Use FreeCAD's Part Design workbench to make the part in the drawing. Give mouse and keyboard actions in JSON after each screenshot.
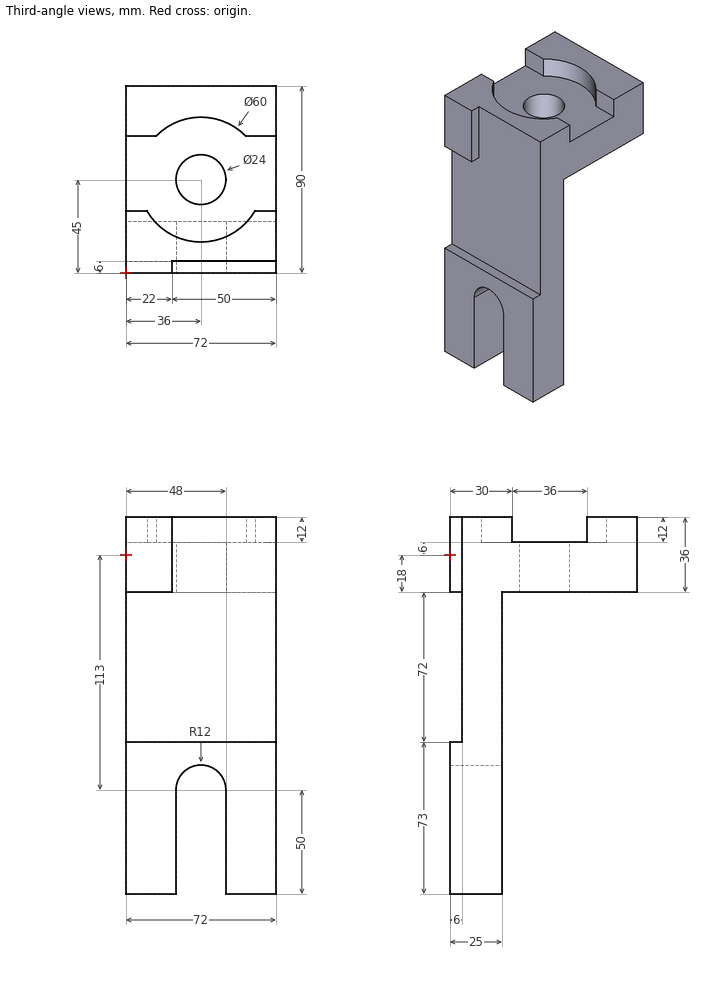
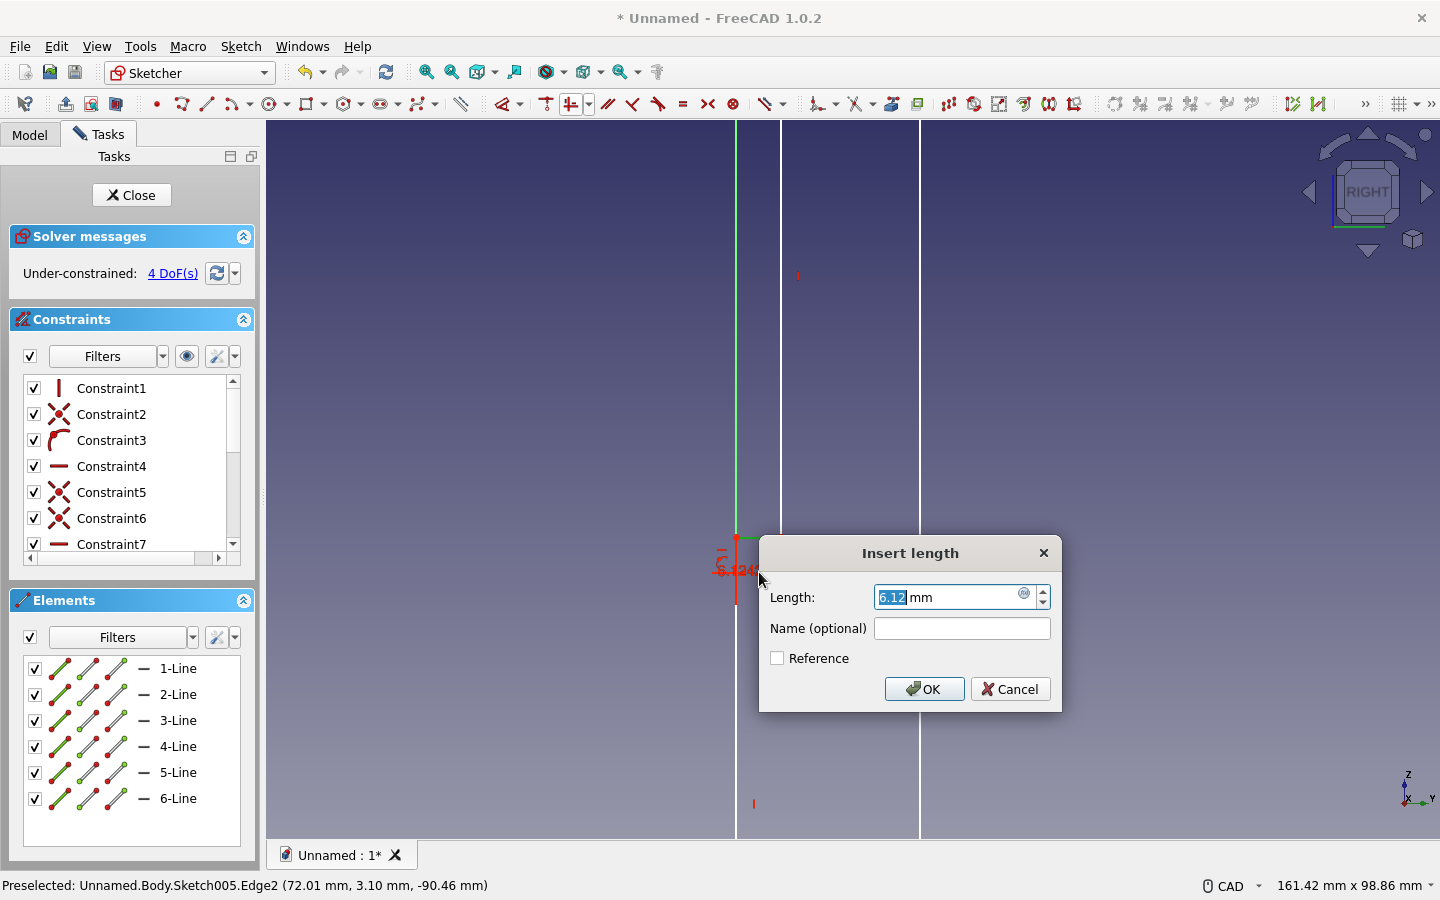
{"action": "type", "text": "6"}
{"action": "key", "text": "Return"}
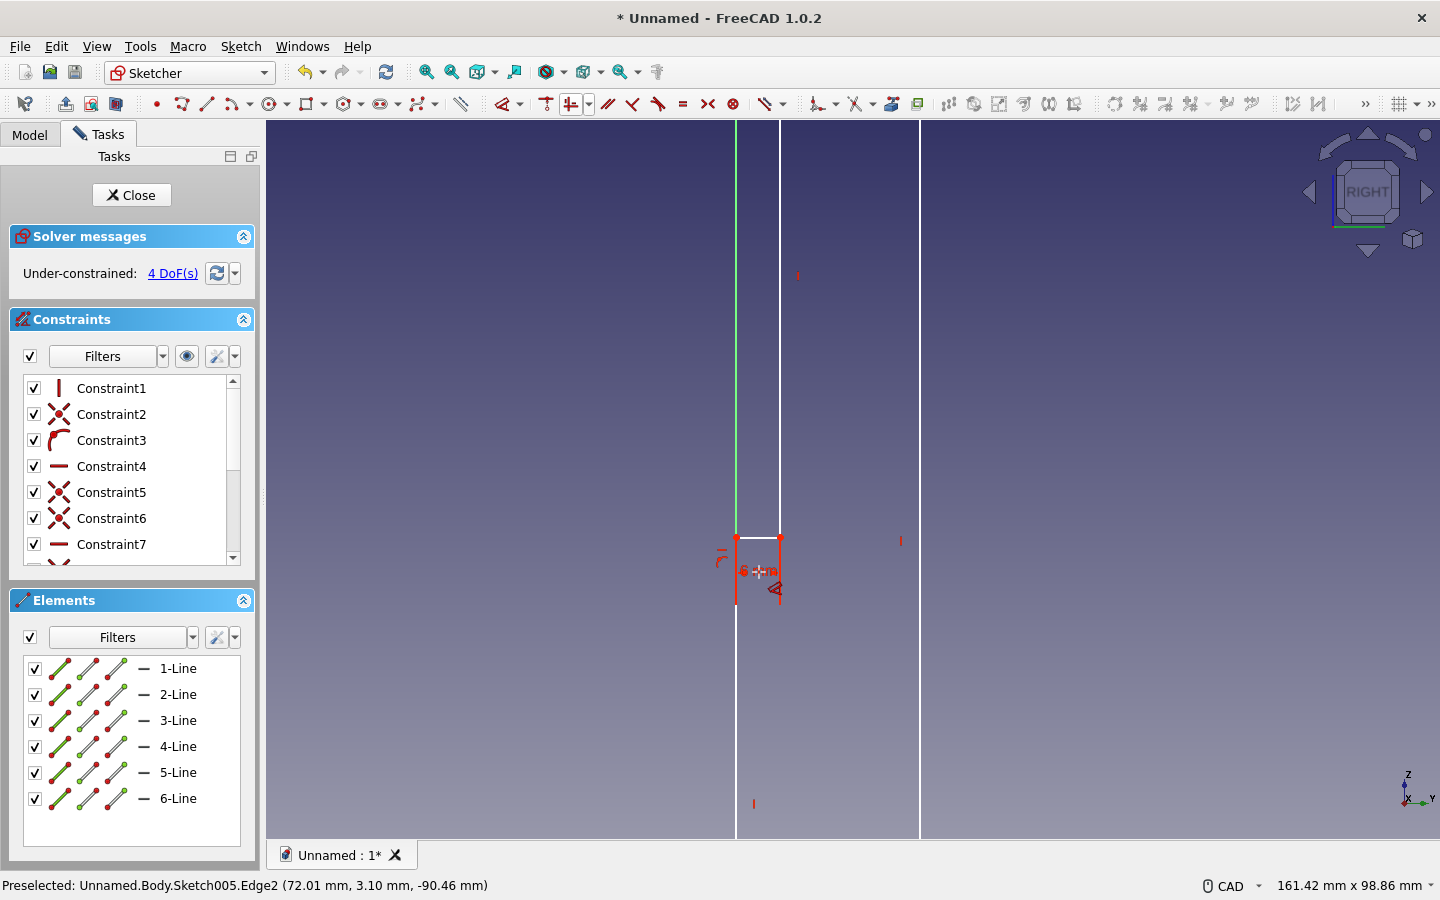
{"action": "left_click", "coordinate": [780, 171]}
{"action": "left_click", "coordinate": [814, 343]}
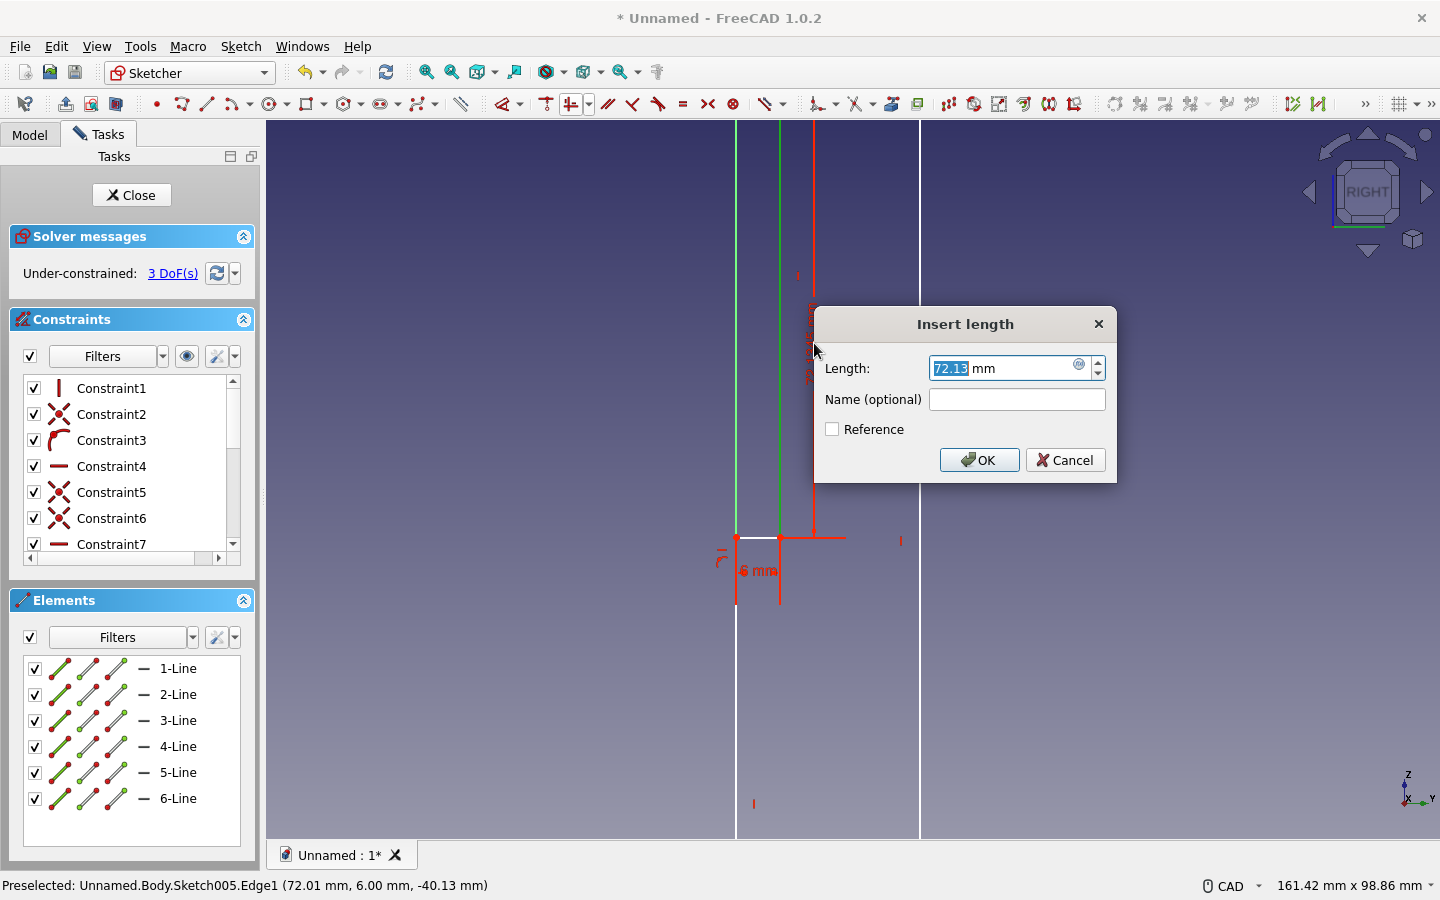
{"action": "type", "text": "72"}
{"action": "key", "text": "Return"}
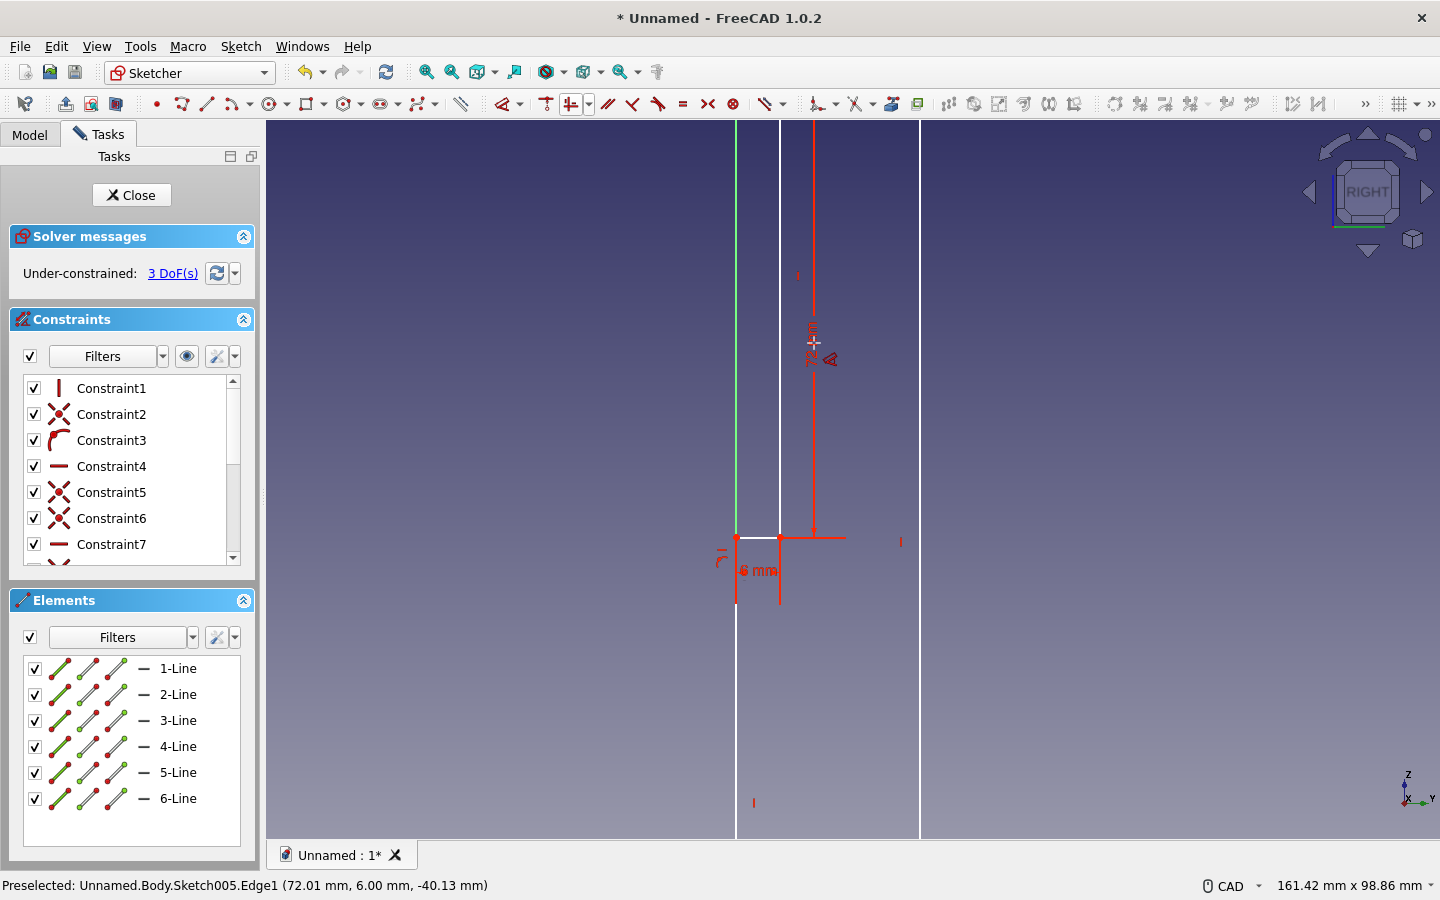
{"action": "left_click", "coordinate": [736, 697]}
{"action": "left_click", "coordinate": [702, 674]}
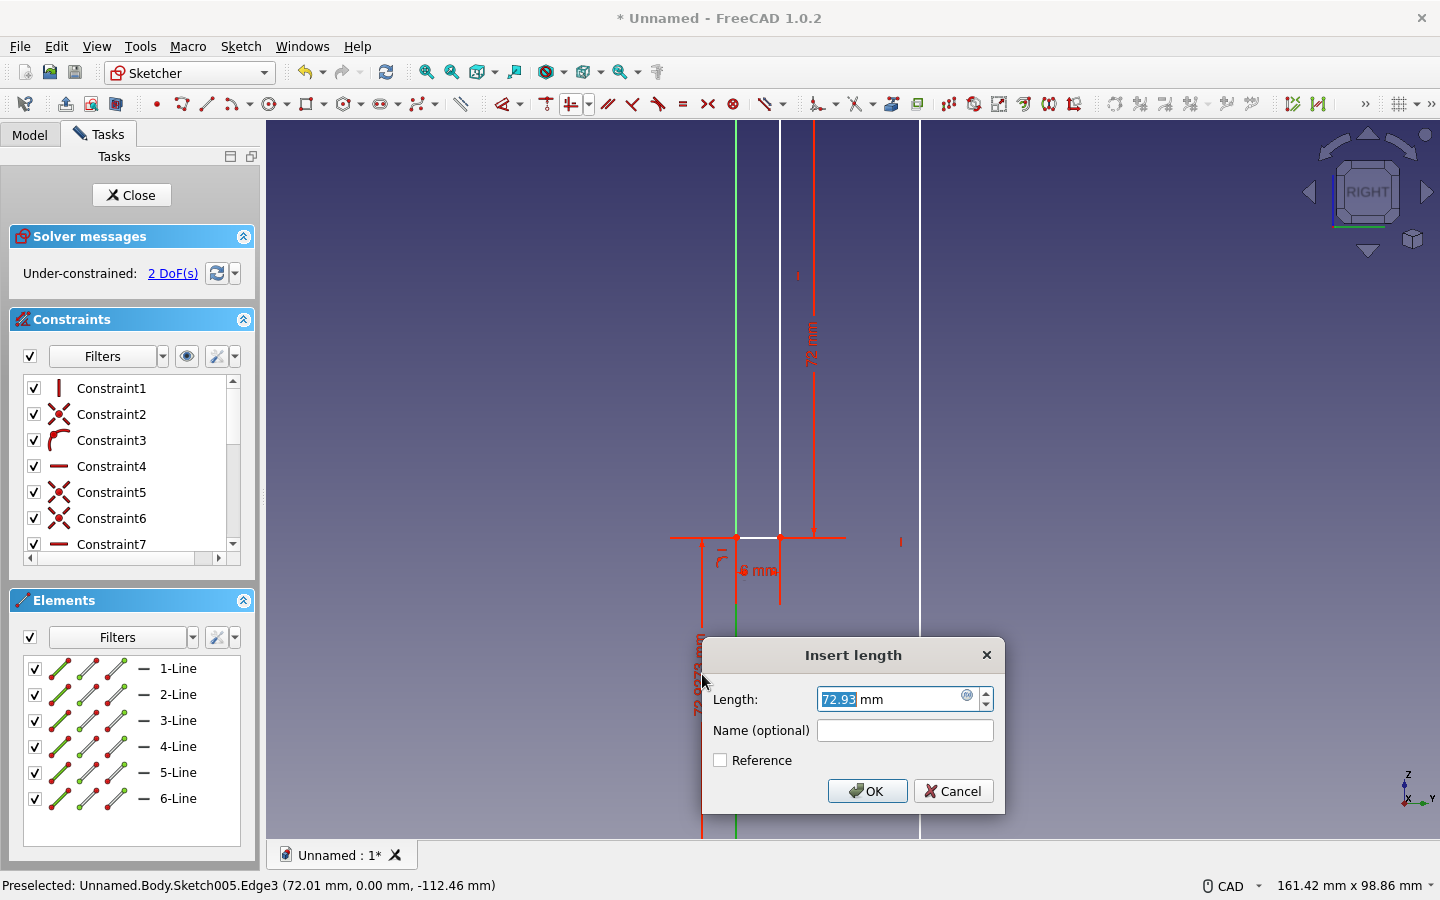
{"action": "type", "text": "73"}
{"action": "key", "text": "Return"}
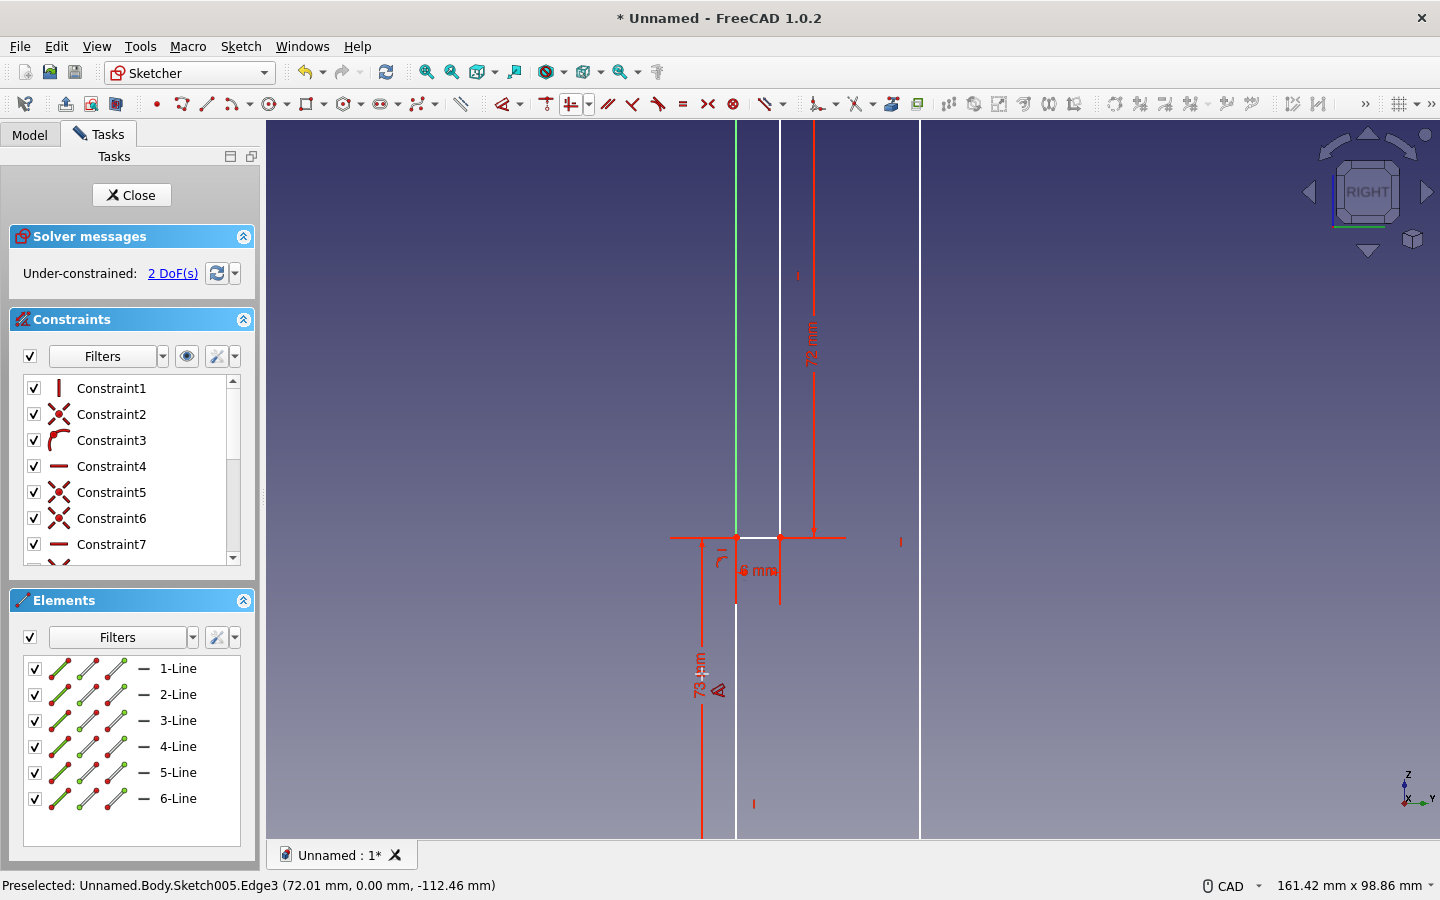
{"action": "scroll", "coordinate": [760, 483], "scroll_direction": "down", "scroll_amount": 5}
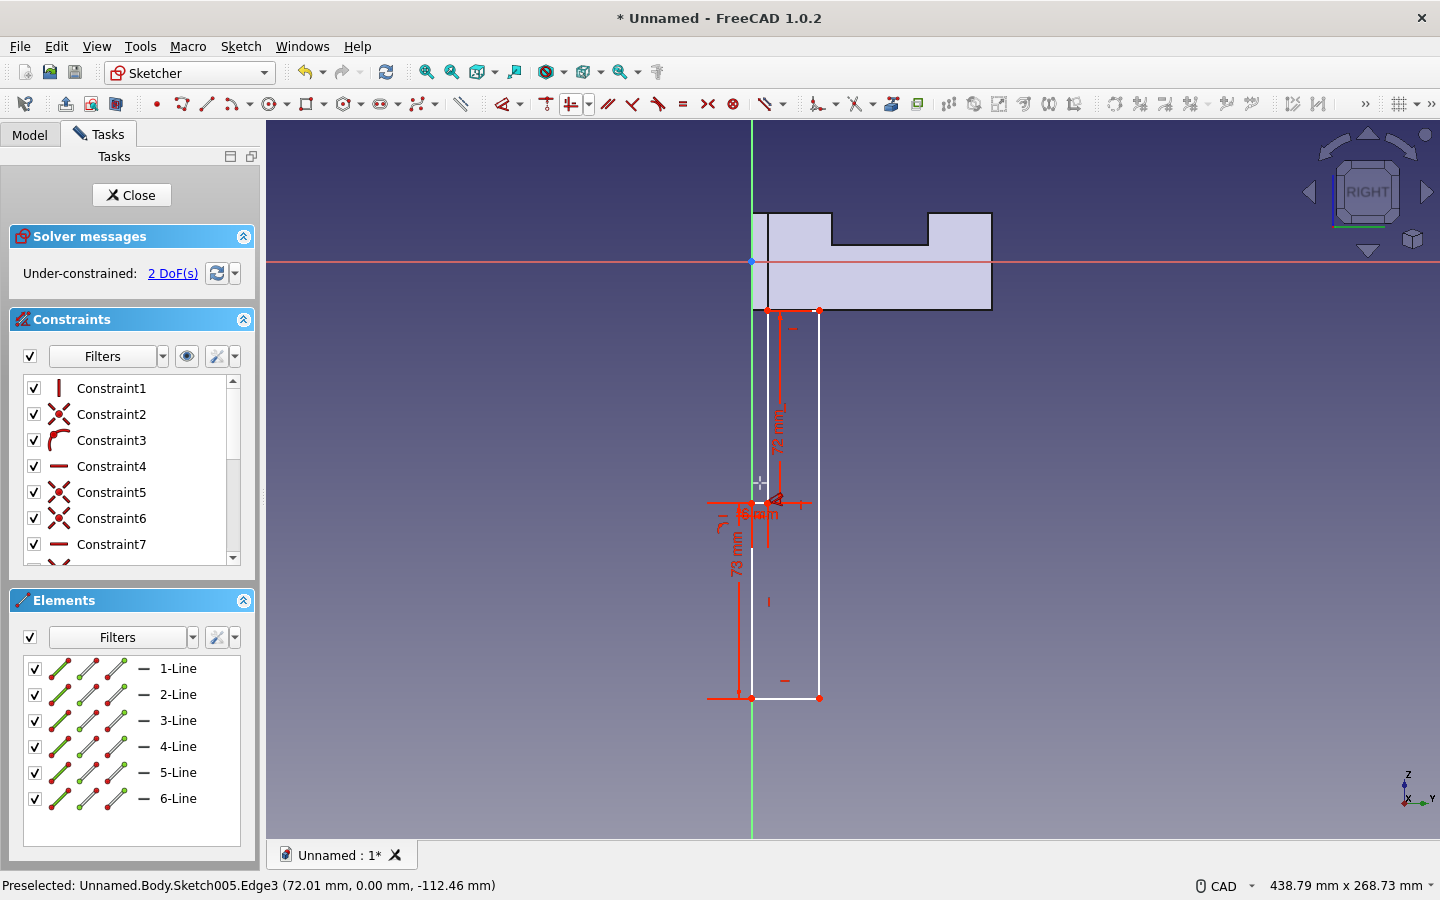
{"action": "left_click", "coordinate": [772, 699]}
{"action": "left_click", "coordinate": [785, 733]}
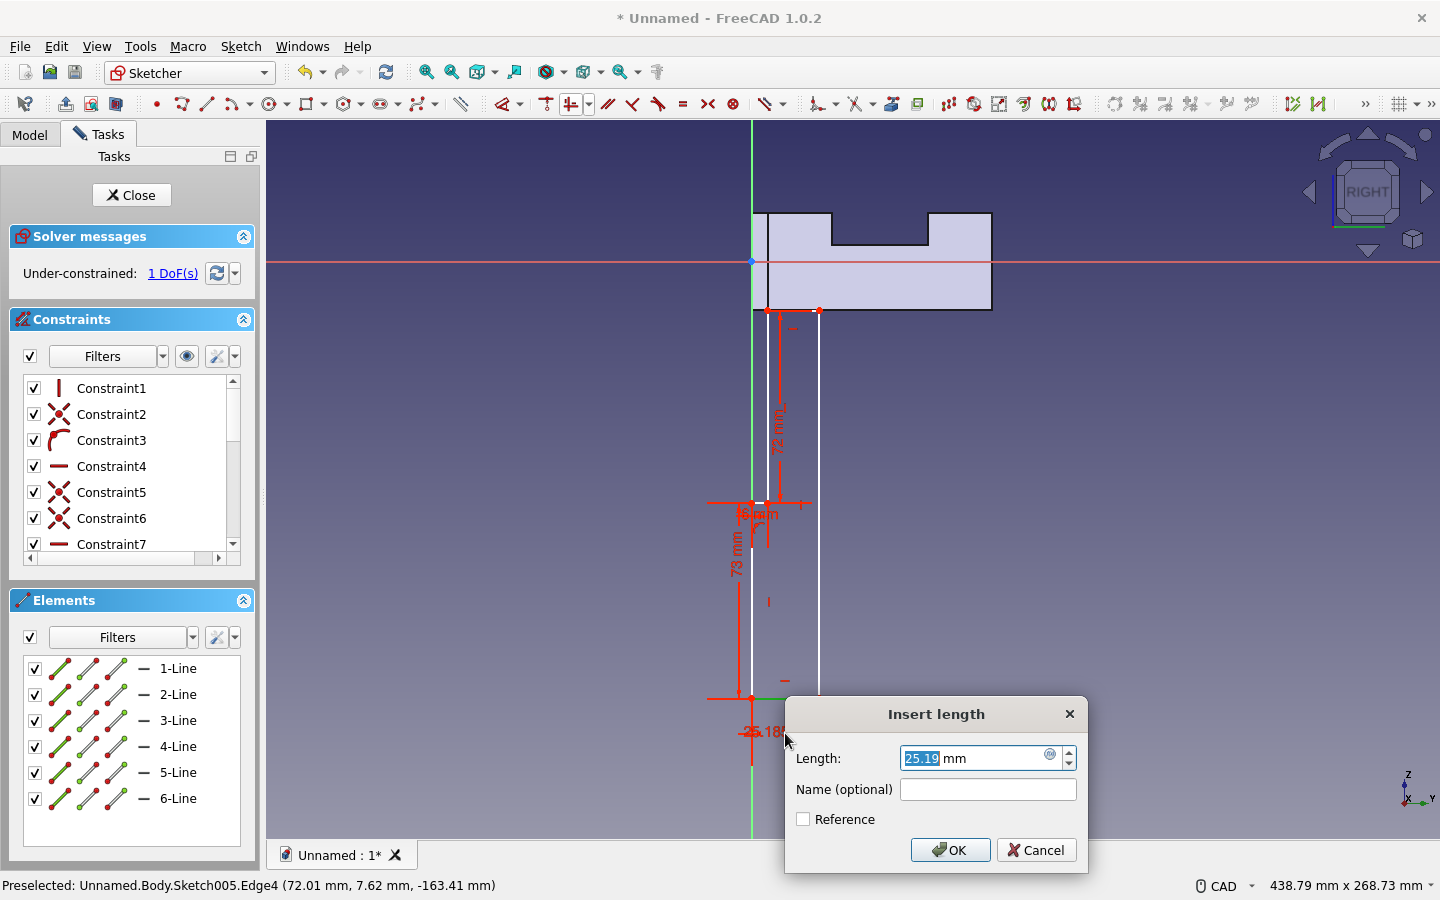
{"action": "type", "text": "25"}
{"action": "key", "text": "Return"}